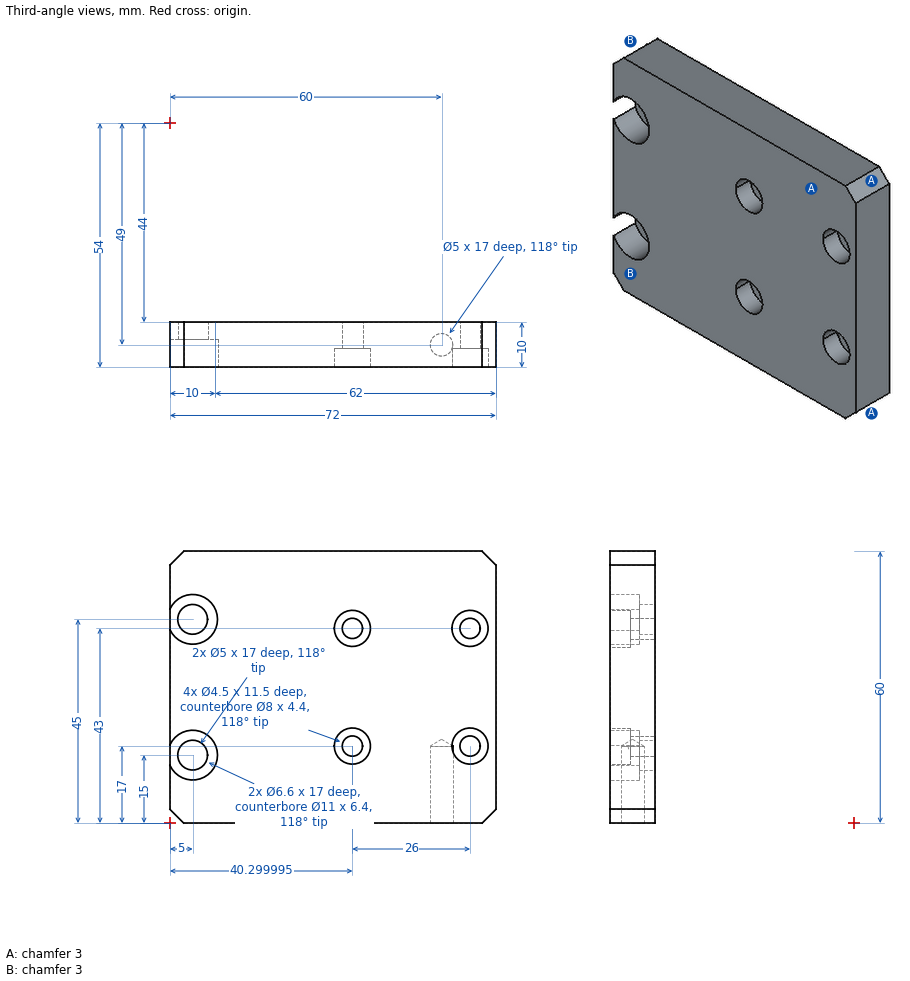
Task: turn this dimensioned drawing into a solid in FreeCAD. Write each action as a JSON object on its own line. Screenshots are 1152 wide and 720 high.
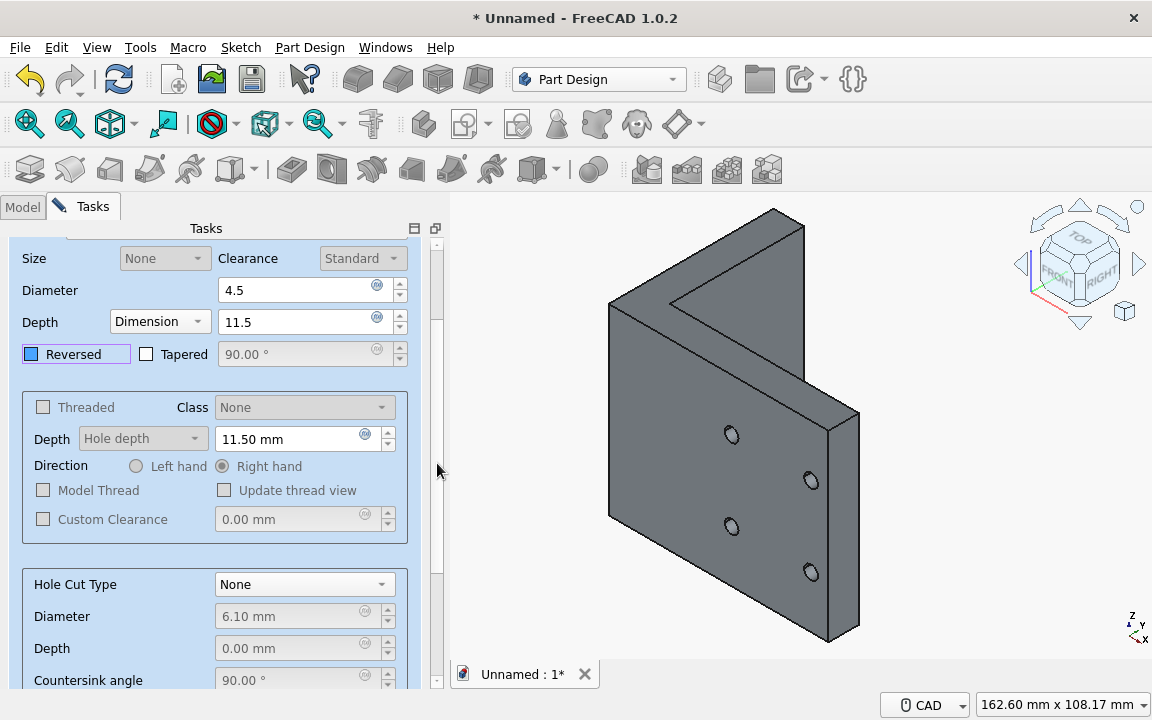
{"action": "left_click", "coordinate": [306, 584]}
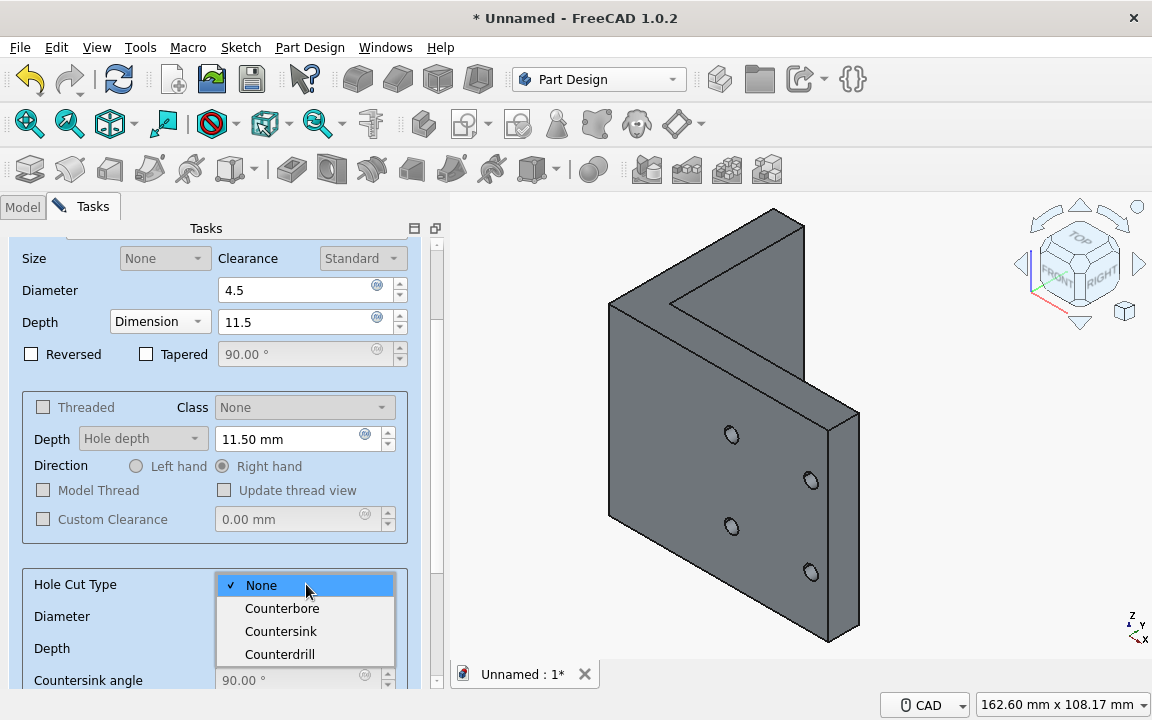
{"action": "left_click", "coordinate": [304, 608]}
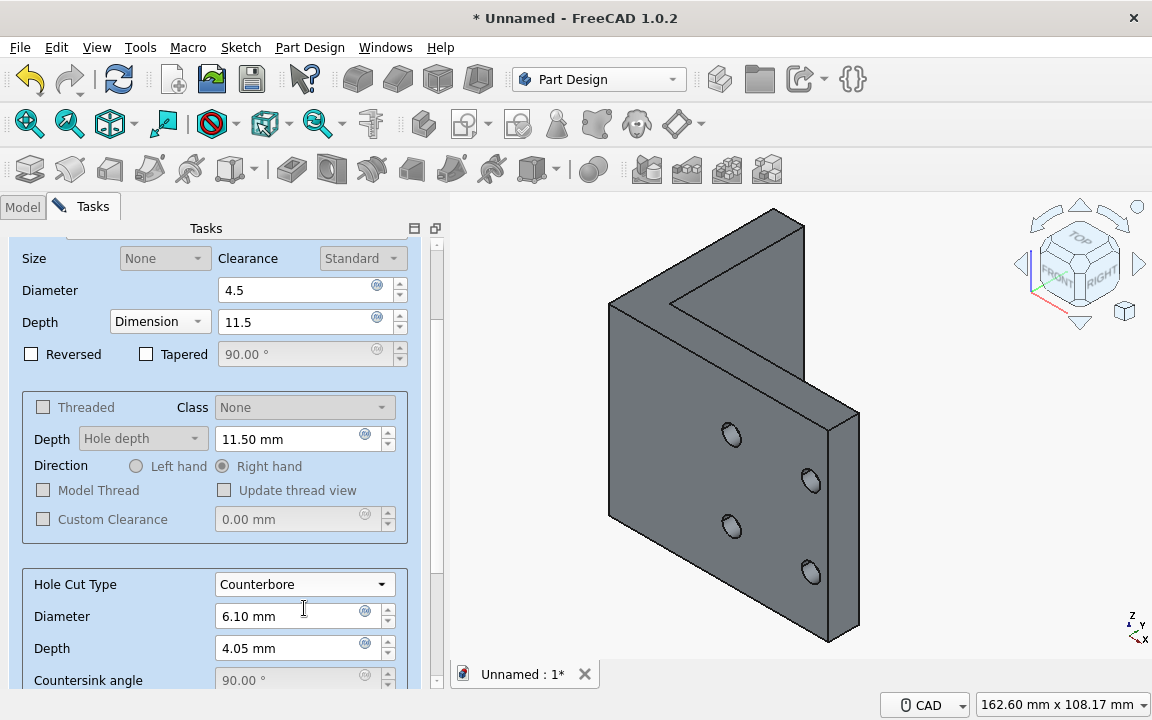
{"action": "triple_click", "coordinate": [298, 616]}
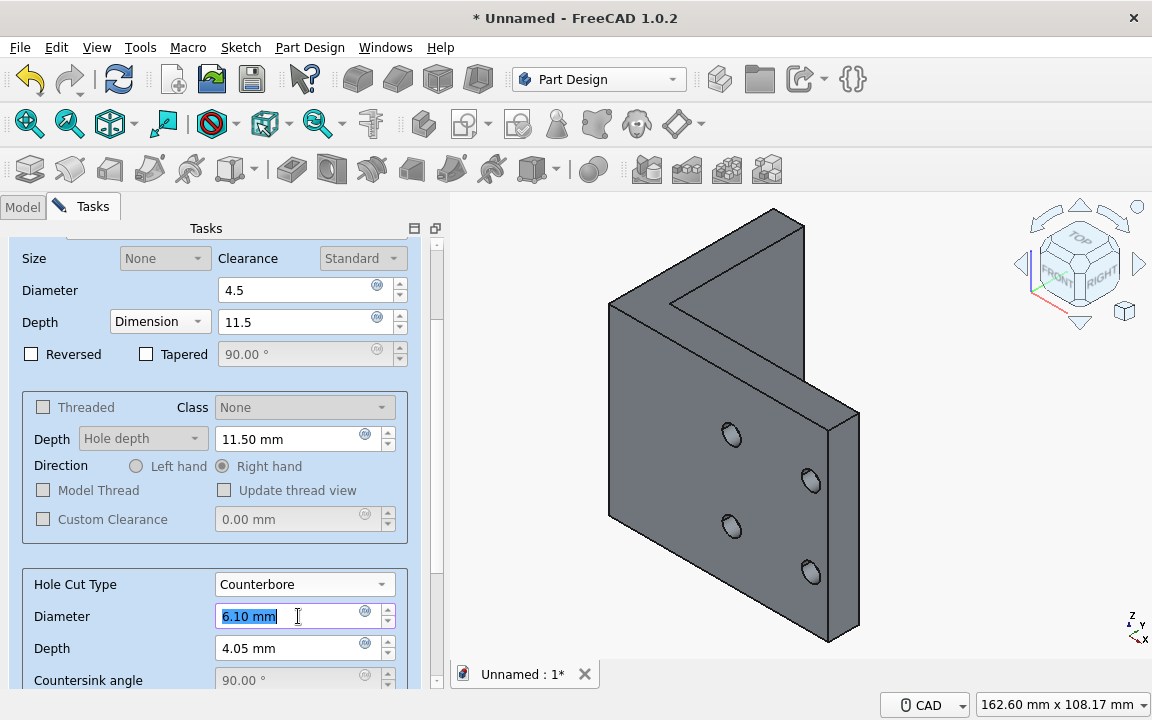
{"action": "type", "text": "8"}
{"action": "key", "text": "Tab"}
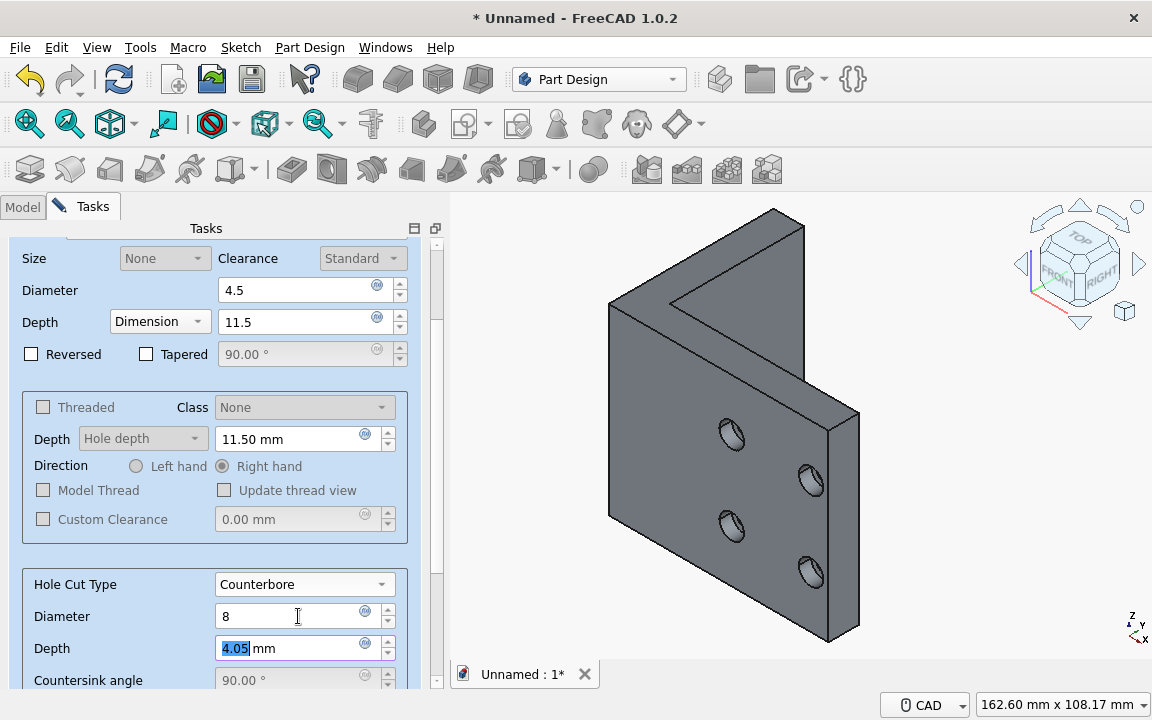
{"action": "type", "text": "4.4"}
{"action": "key", "text": "Tab"}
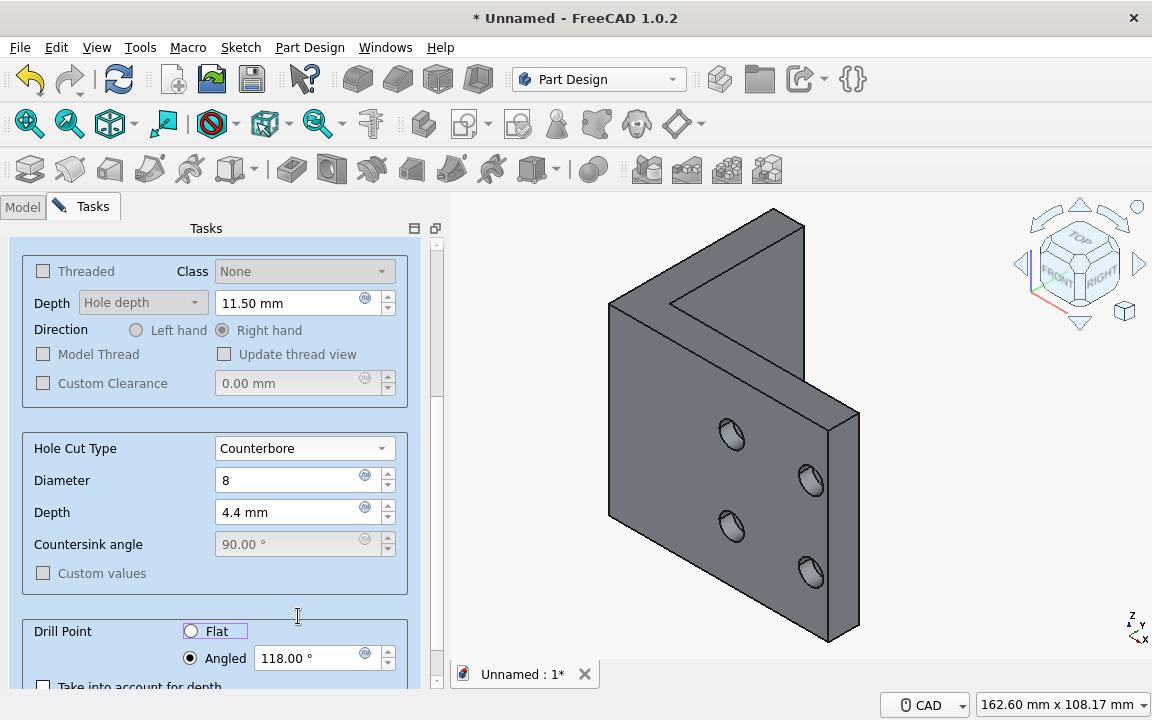
{"action": "scroll", "coordinate": [437, 463], "scroll_direction": "up", "scroll_amount": 6}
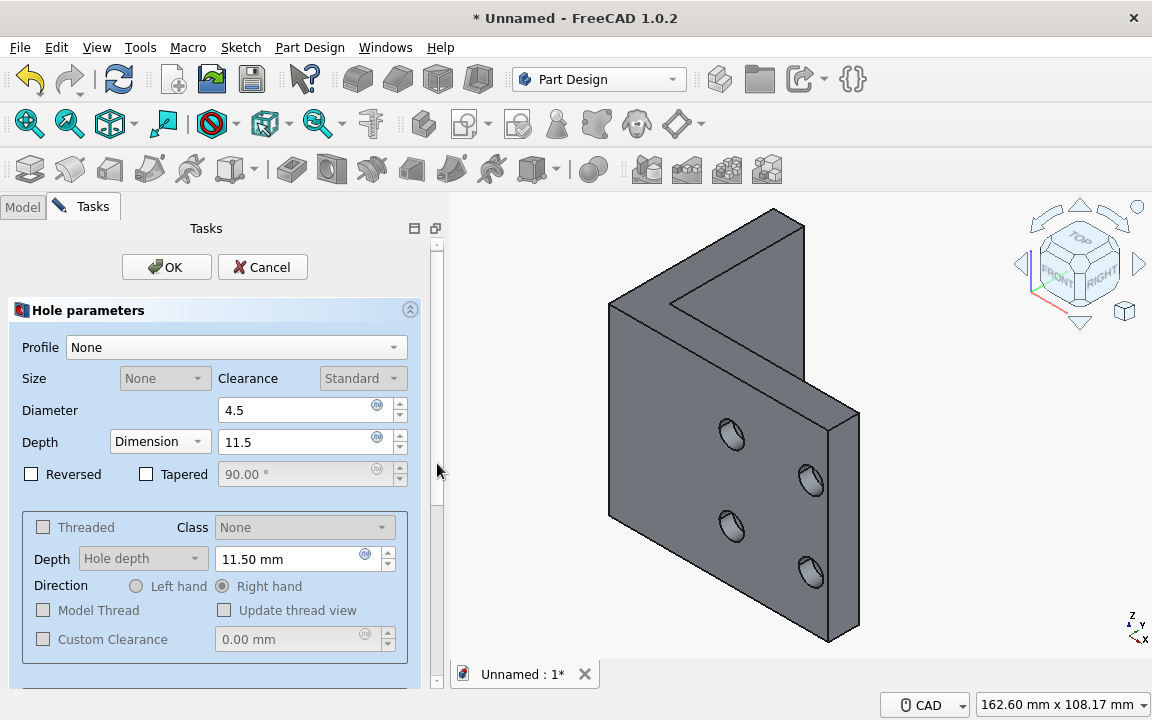
{"action": "left_click", "coordinate": [167, 267]}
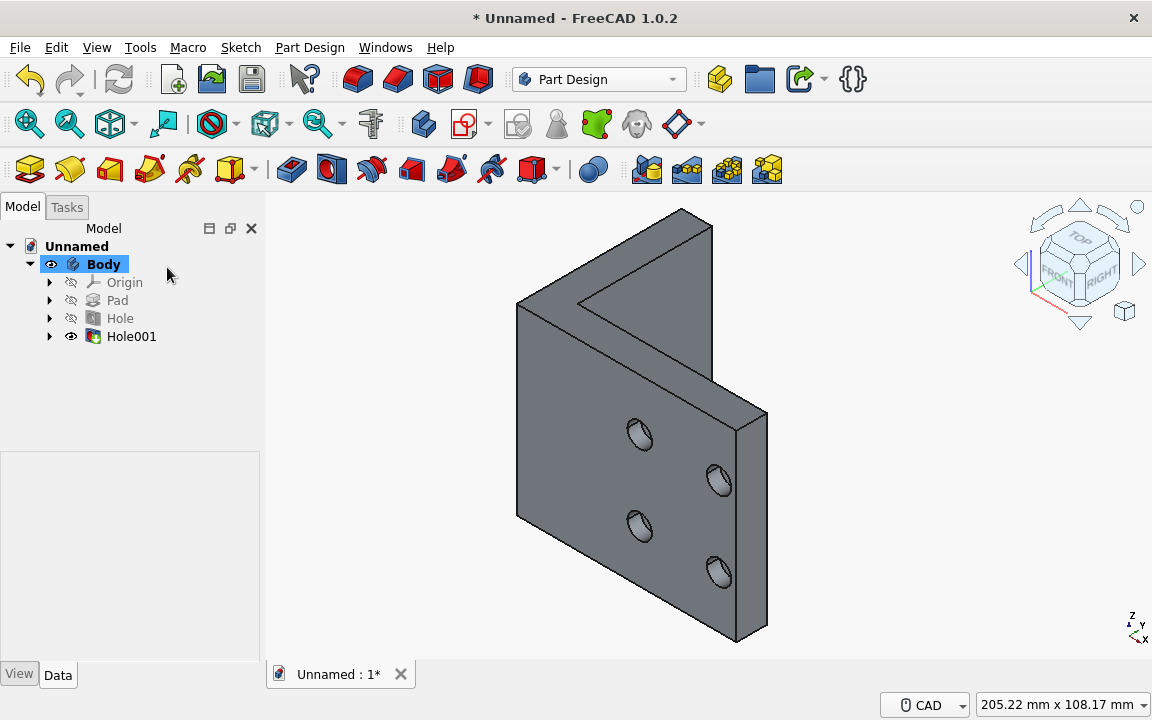
{"action": "key", "text": "4"}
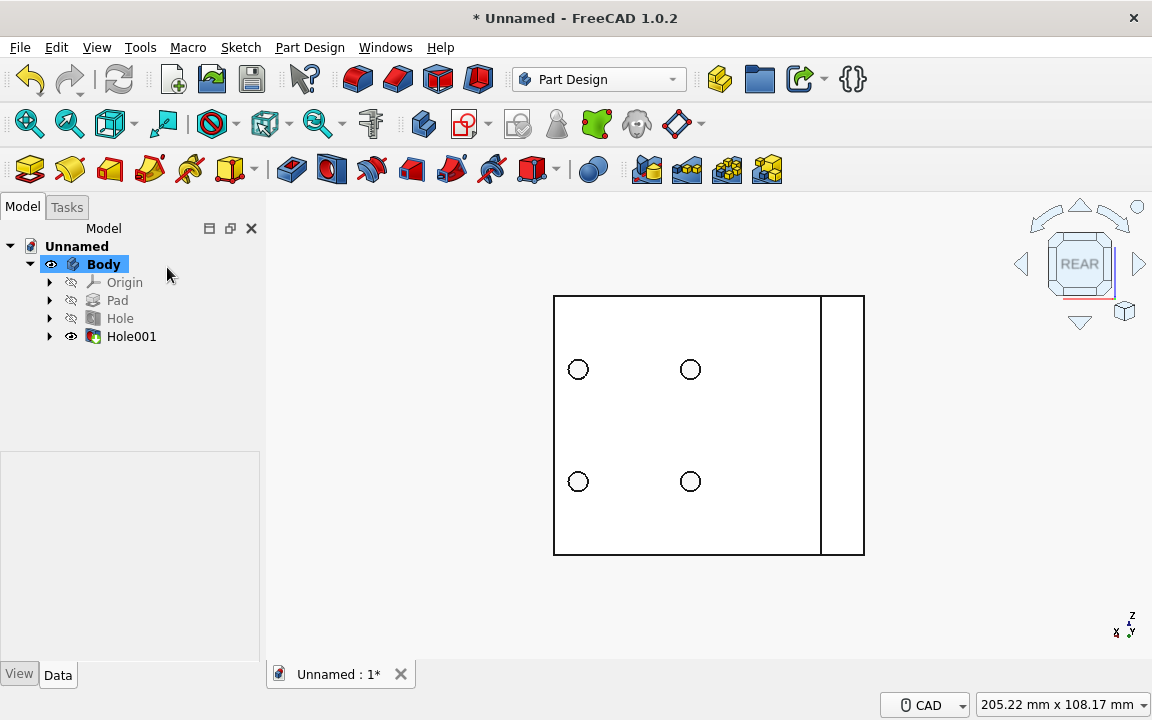
{"action": "left_click", "coordinate": [843, 350]}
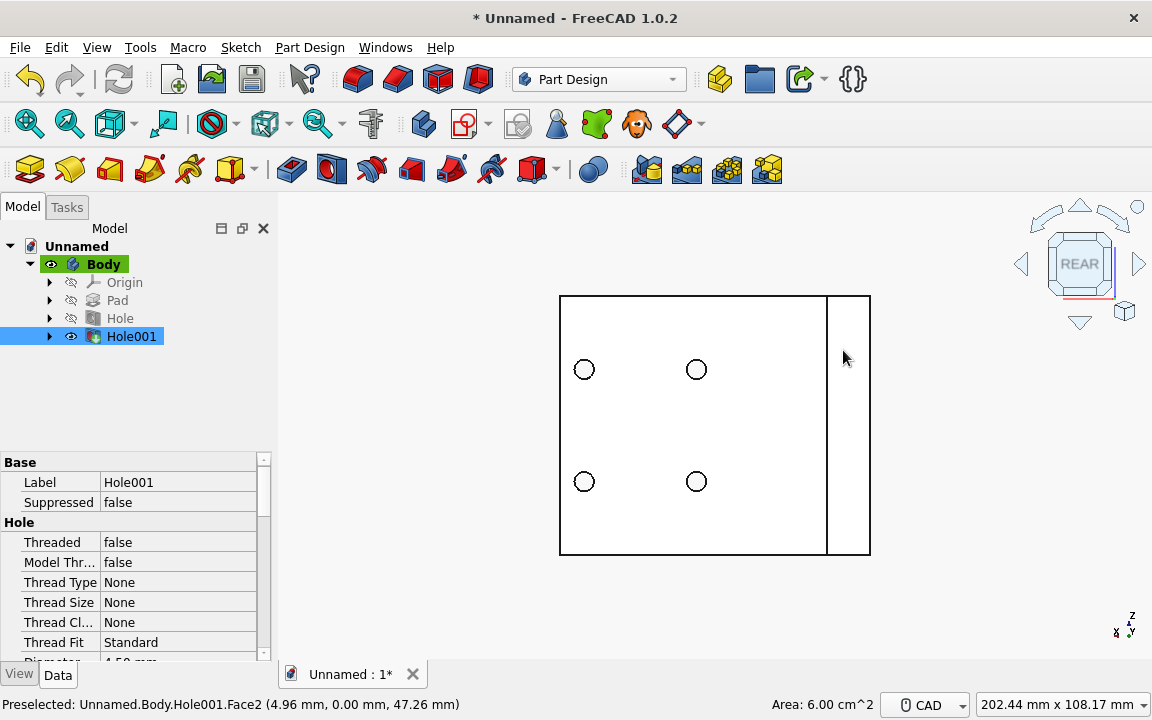
{"action": "left_click", "coordinate": [464, 124]}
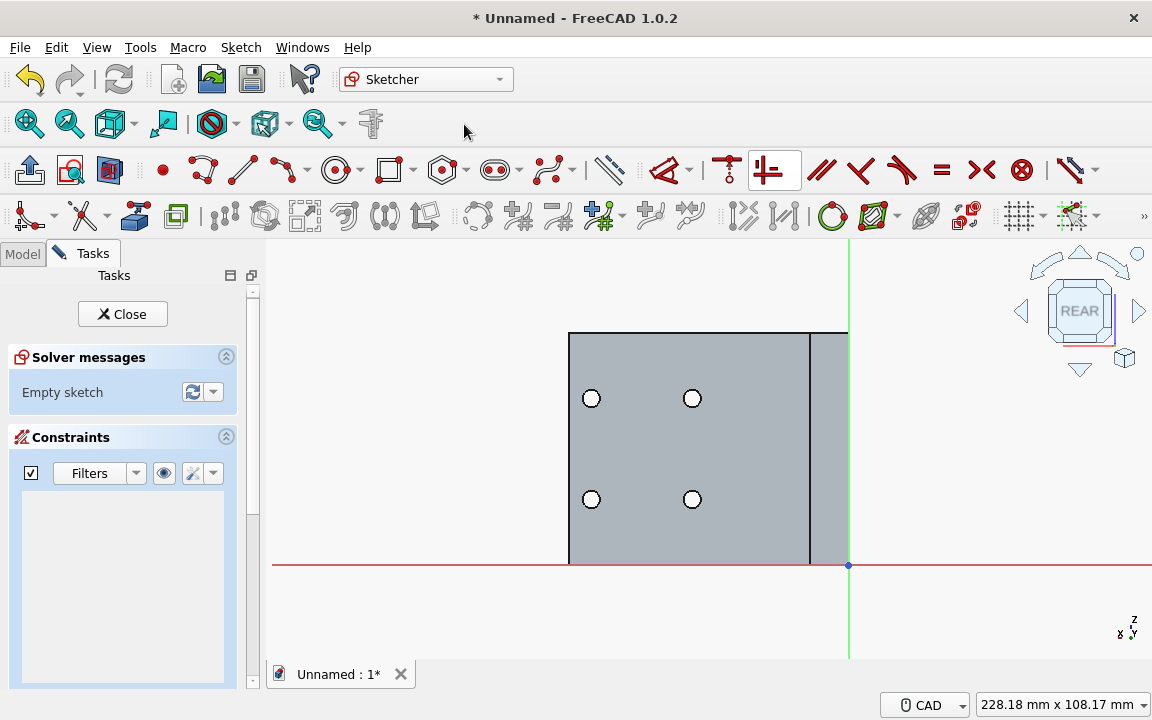
{"action": "scroll", "coordinate": [987, 523], "scroll_direction": "up", "scroll_amount": 2}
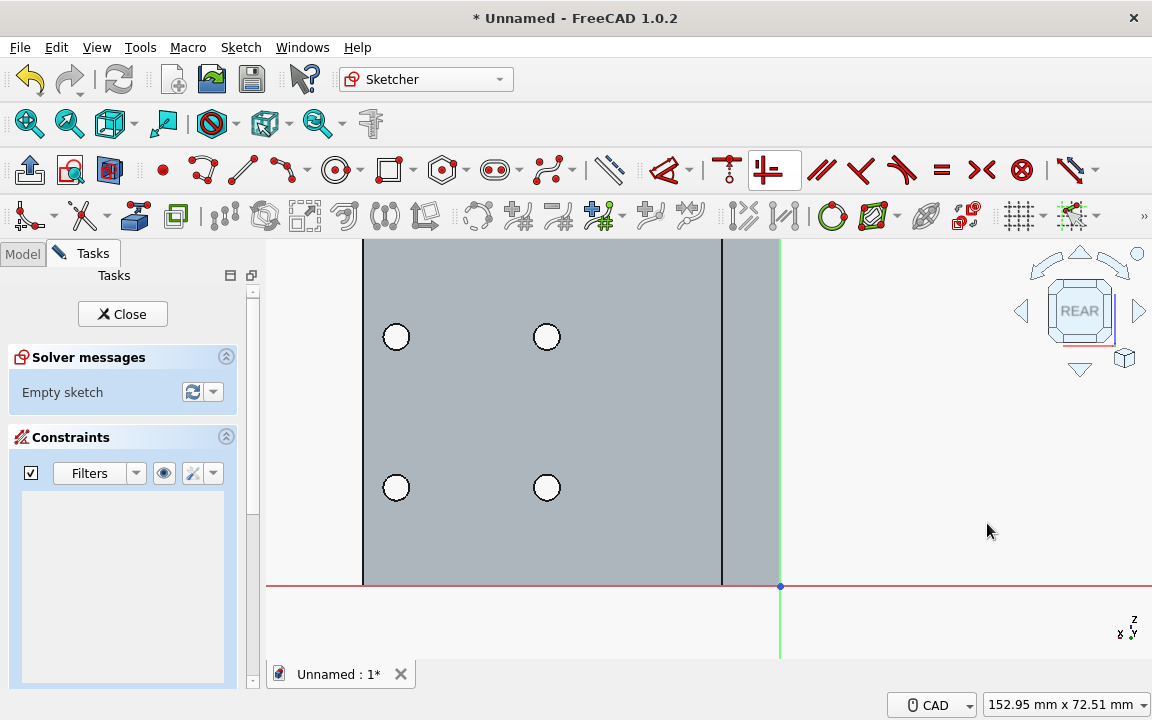
{"action": "left_click", "coordinate": [336, 170]}